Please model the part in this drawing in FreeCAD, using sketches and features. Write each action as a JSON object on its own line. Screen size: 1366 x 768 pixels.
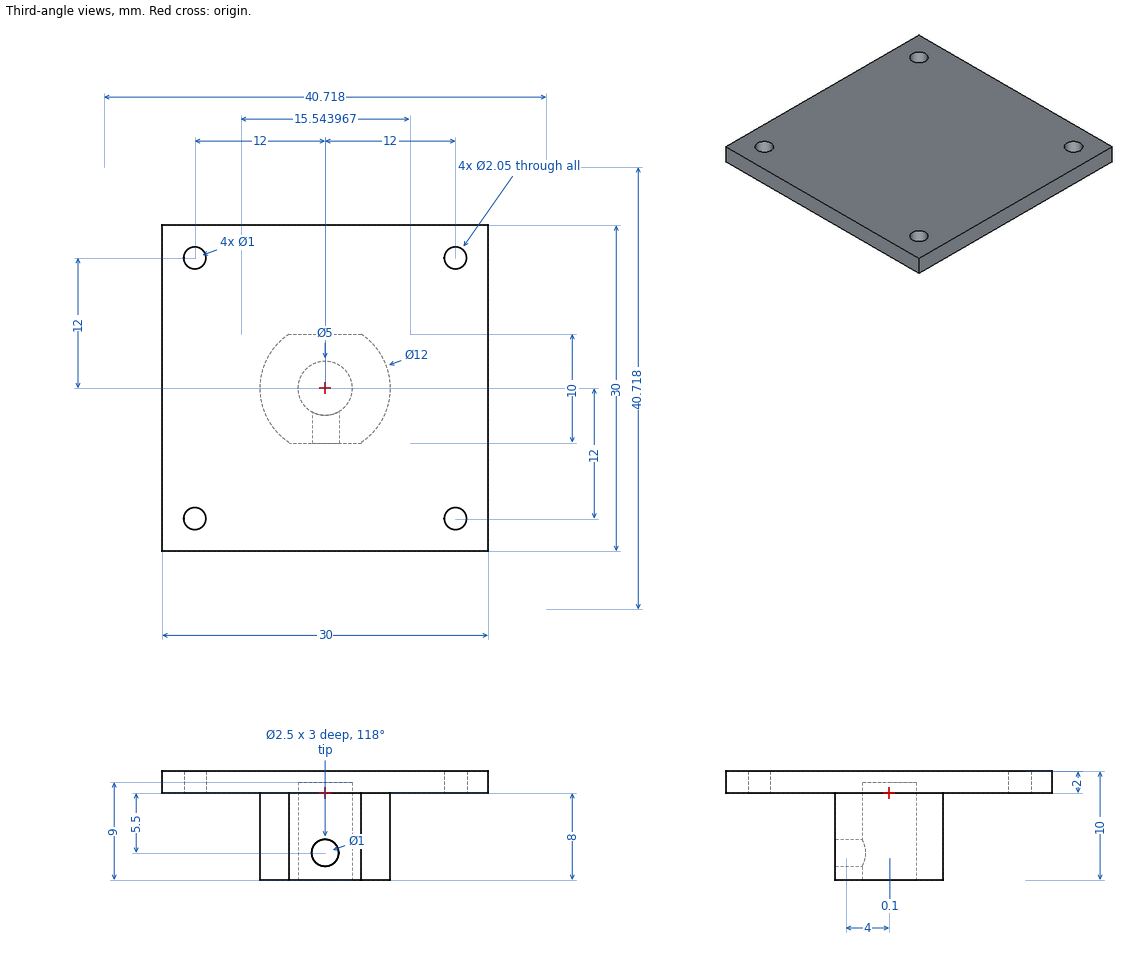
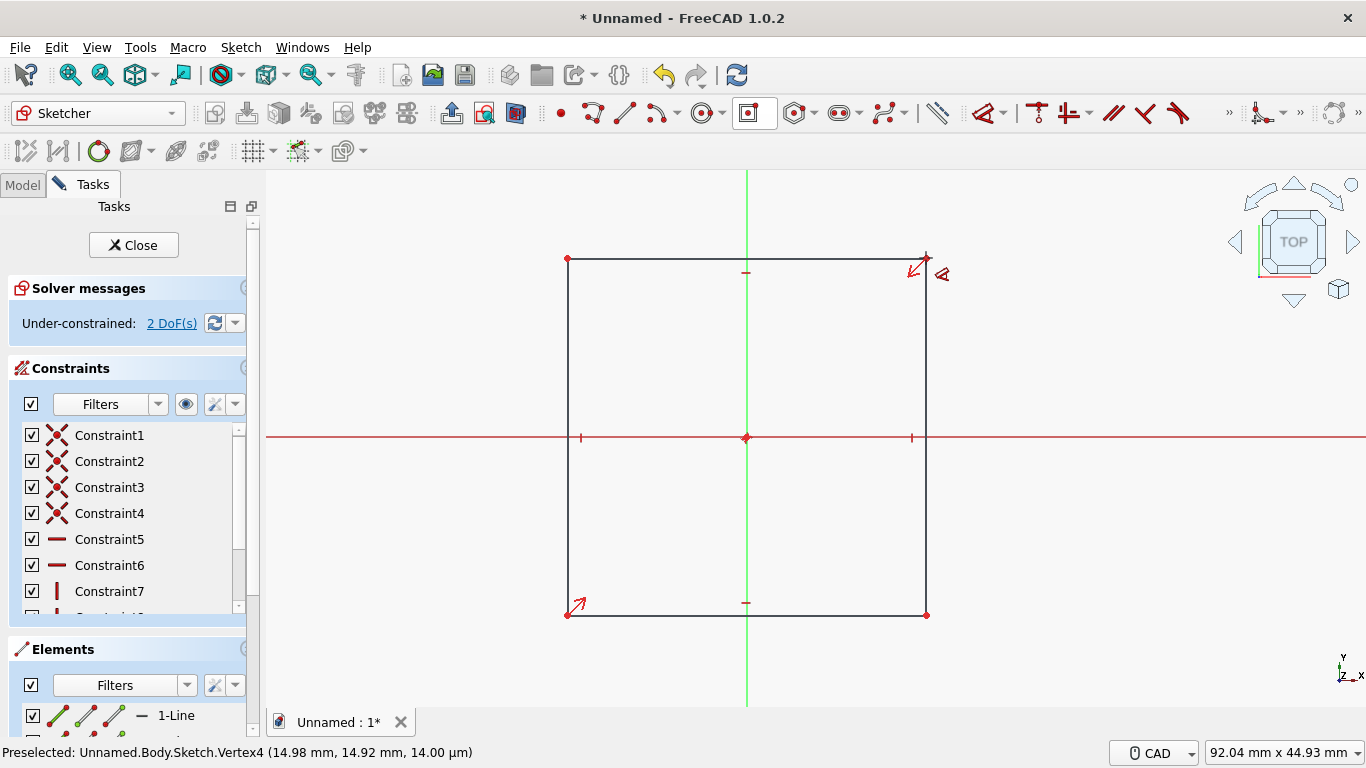
{"action": "left_click", "coordinate": [675, 616]}
{"action": "left_click", "coordinate": [665, 650]}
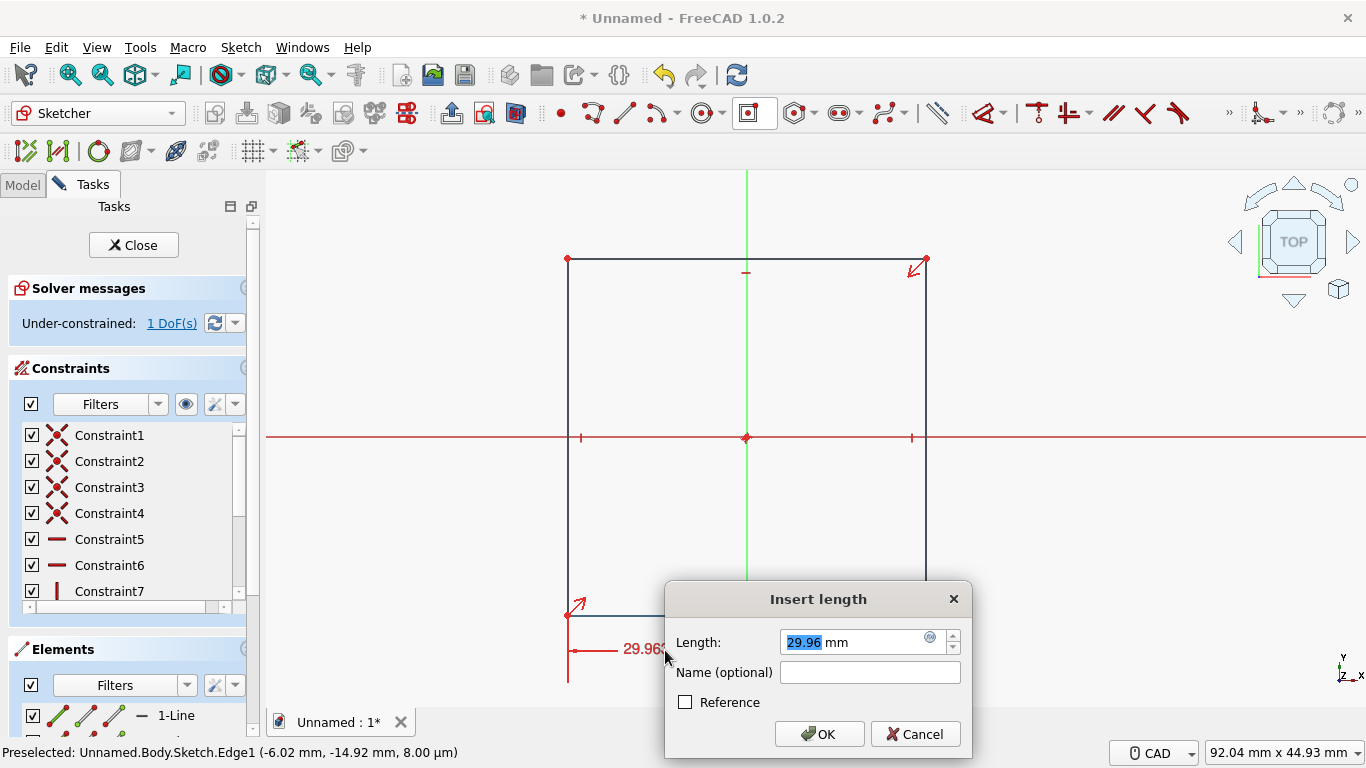
{"action": "type", "text": "30"}
{"action": "key", "text": "Return"}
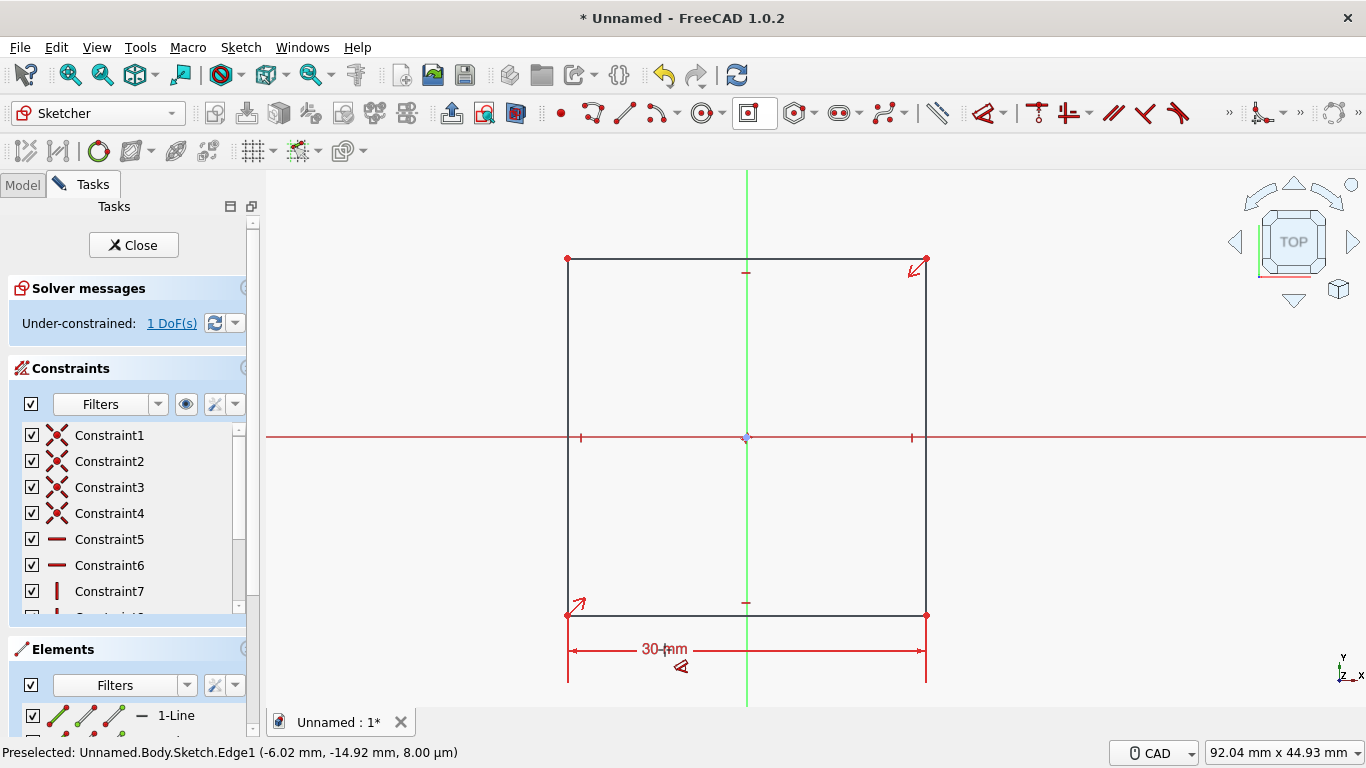
{"action": "left_click", "coordinate": [926, 509]}
{"action": "left_click", "coordinate": [960, 355]}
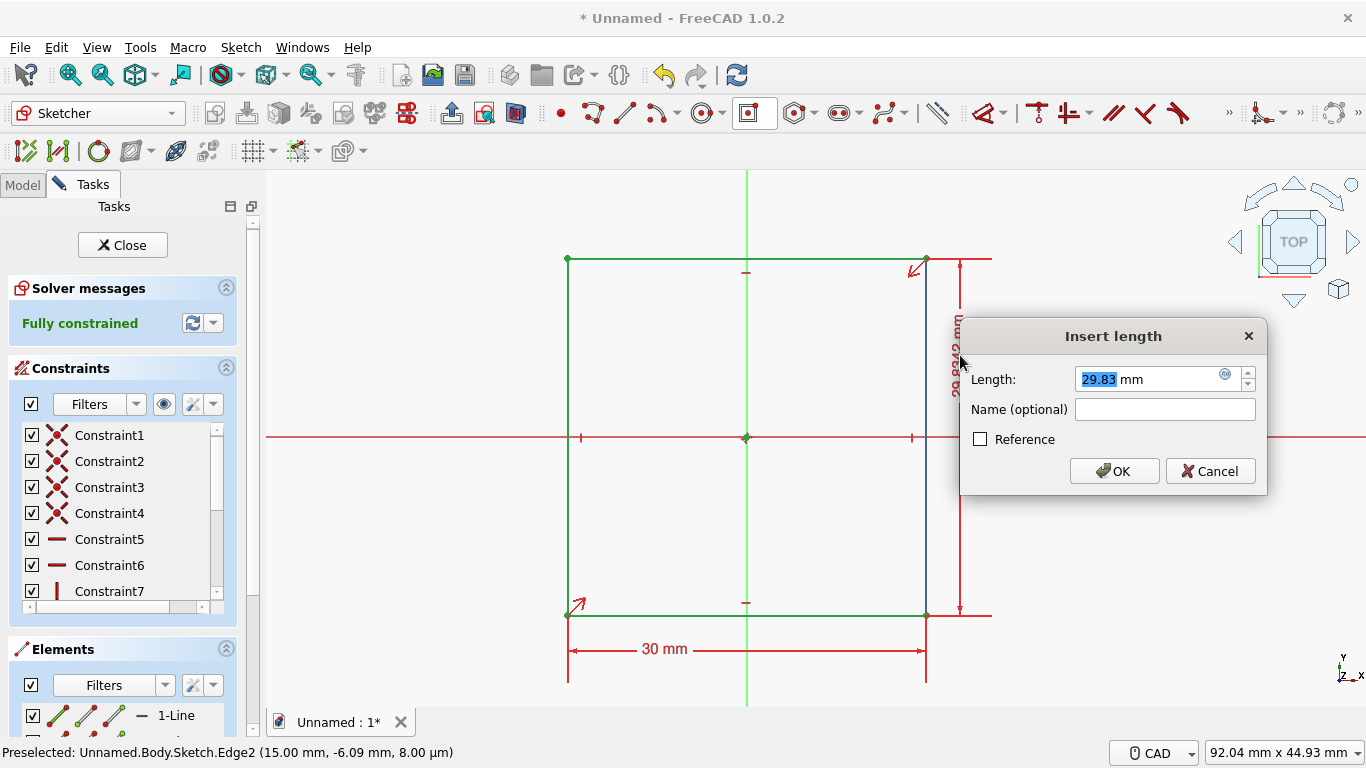
{"action": "type", "text": "30"}
{"action": "key", "text": "Return"}
{"action": "key", "text": "Escape"}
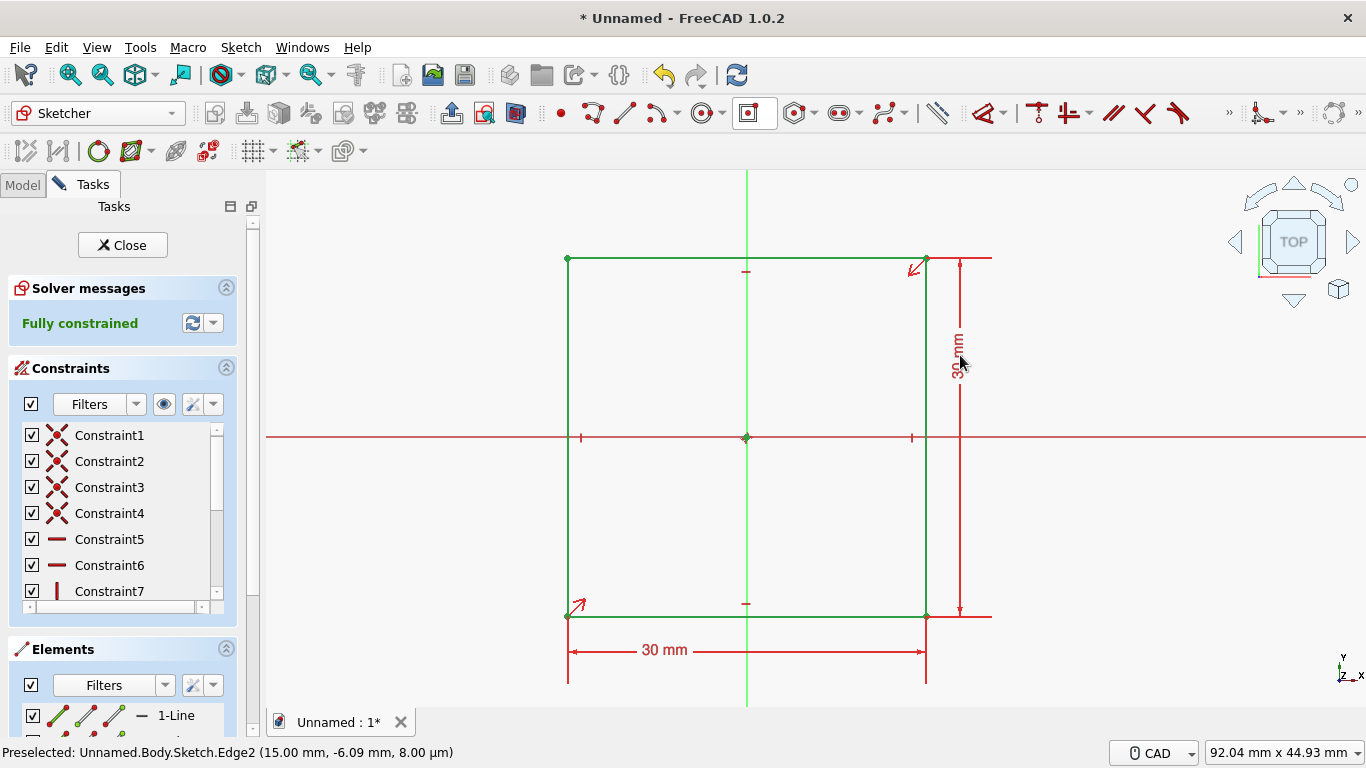
{"action": "left_click", "coordinate": [123, 245]}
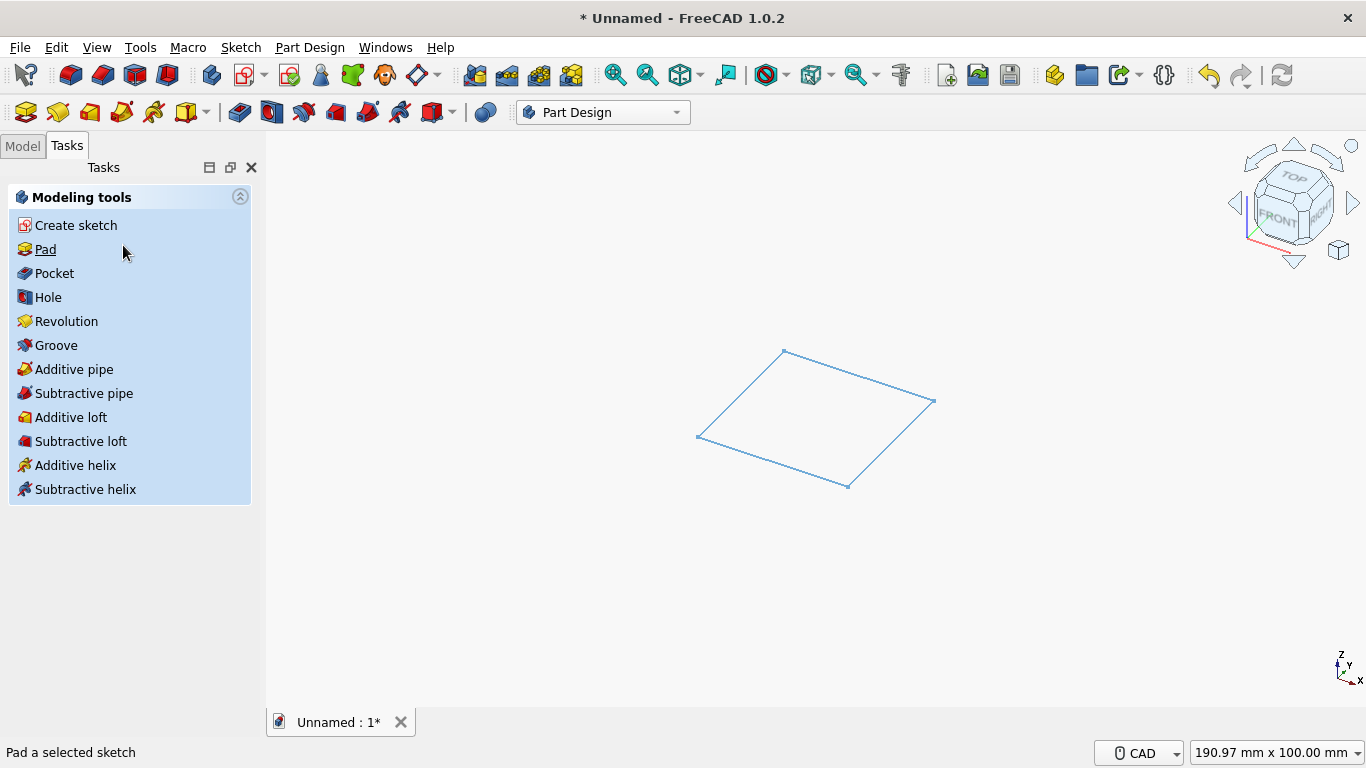
{"action": "left_click", "coordinate": [26, 112]}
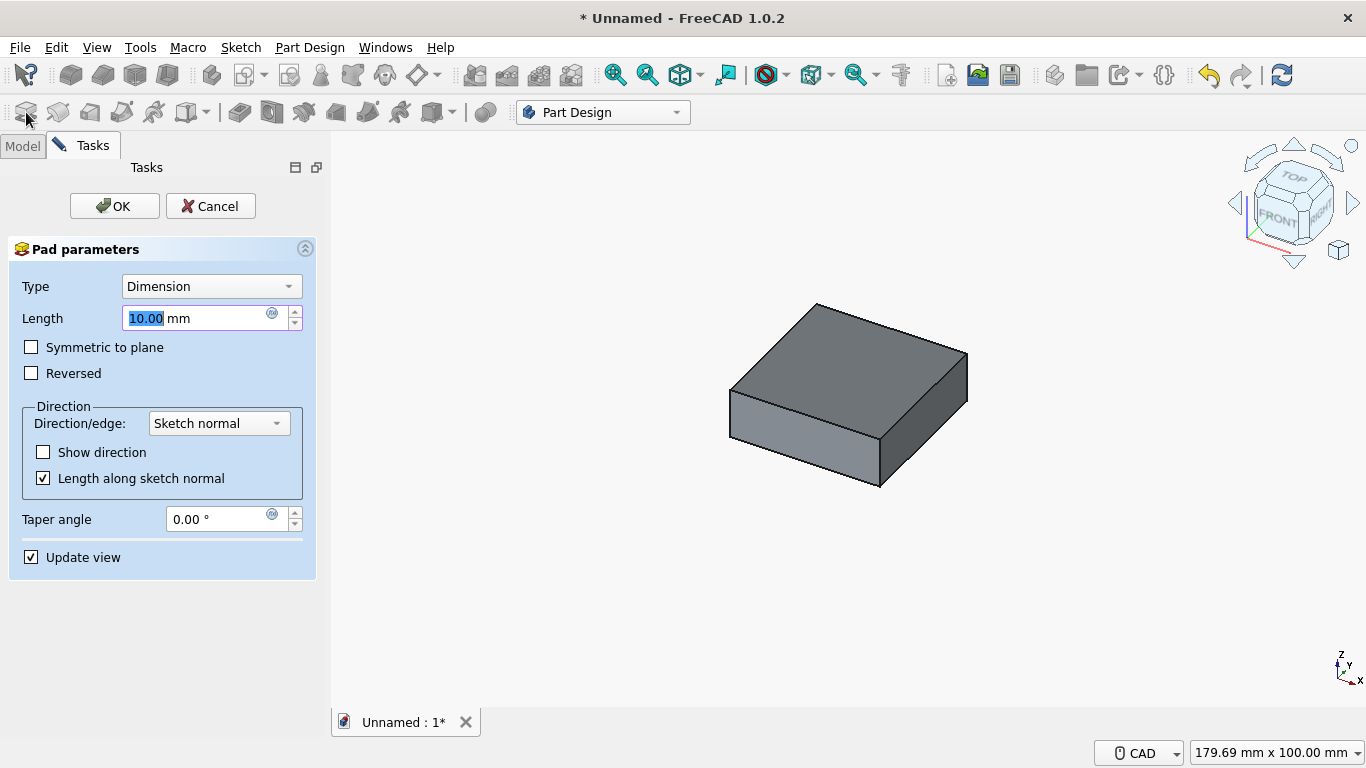
{"action": "type", "text": "2"}
{"action": "key", "text": "Tab"}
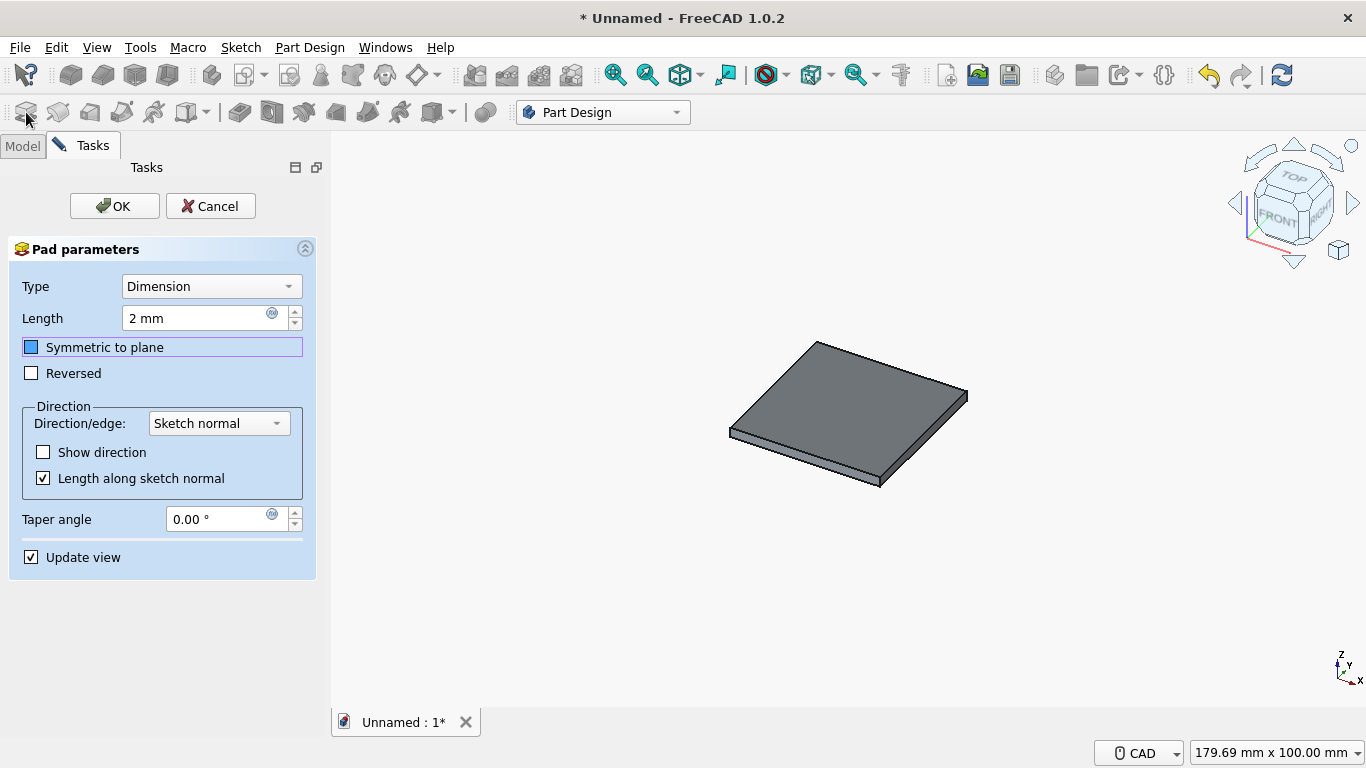
{"action": "left_click", "coordinate": [115, 206]}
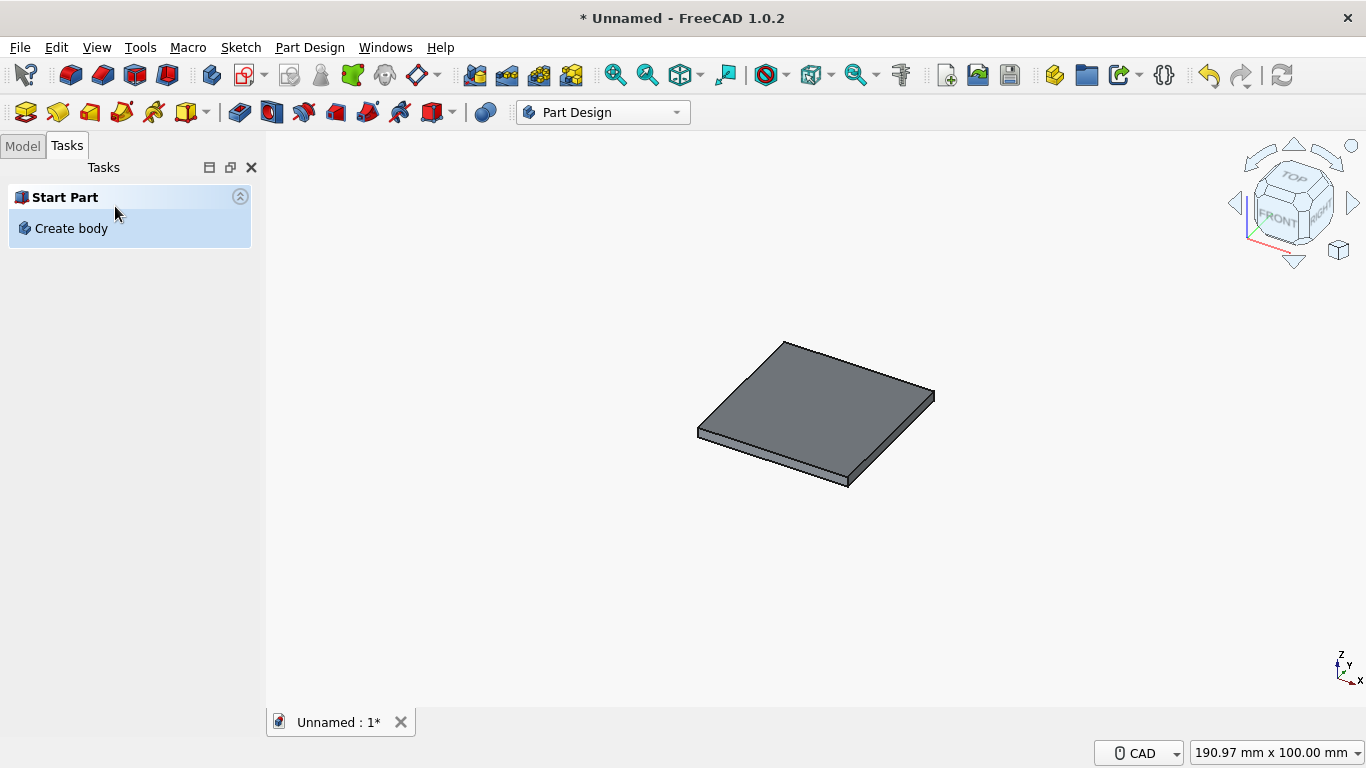
{"action": "key", "text": "v f"}